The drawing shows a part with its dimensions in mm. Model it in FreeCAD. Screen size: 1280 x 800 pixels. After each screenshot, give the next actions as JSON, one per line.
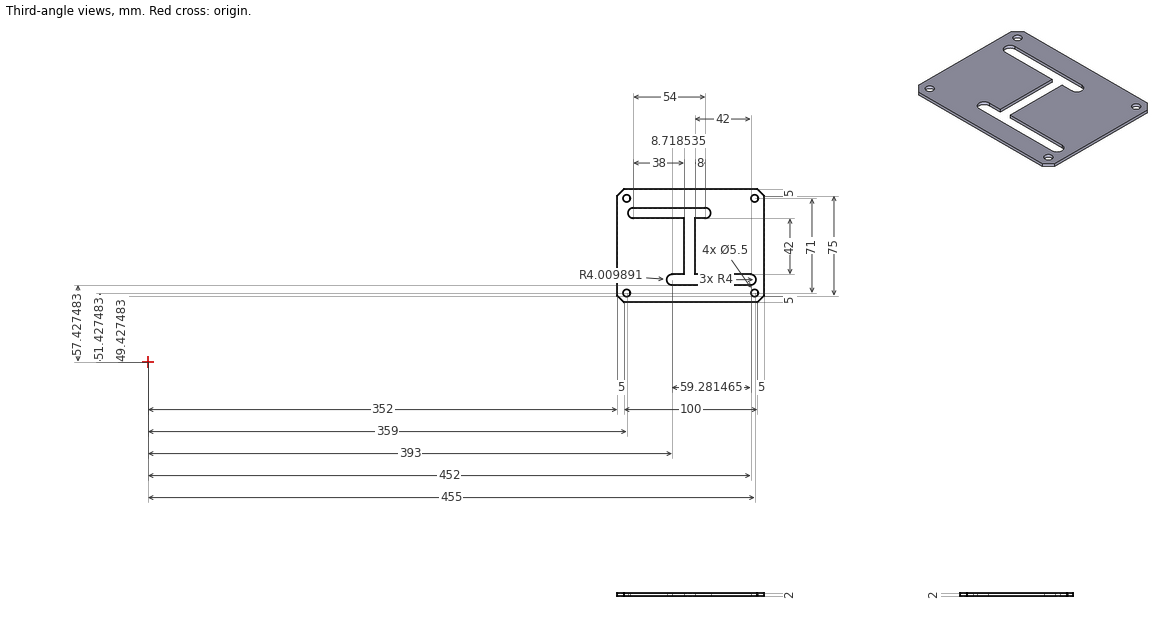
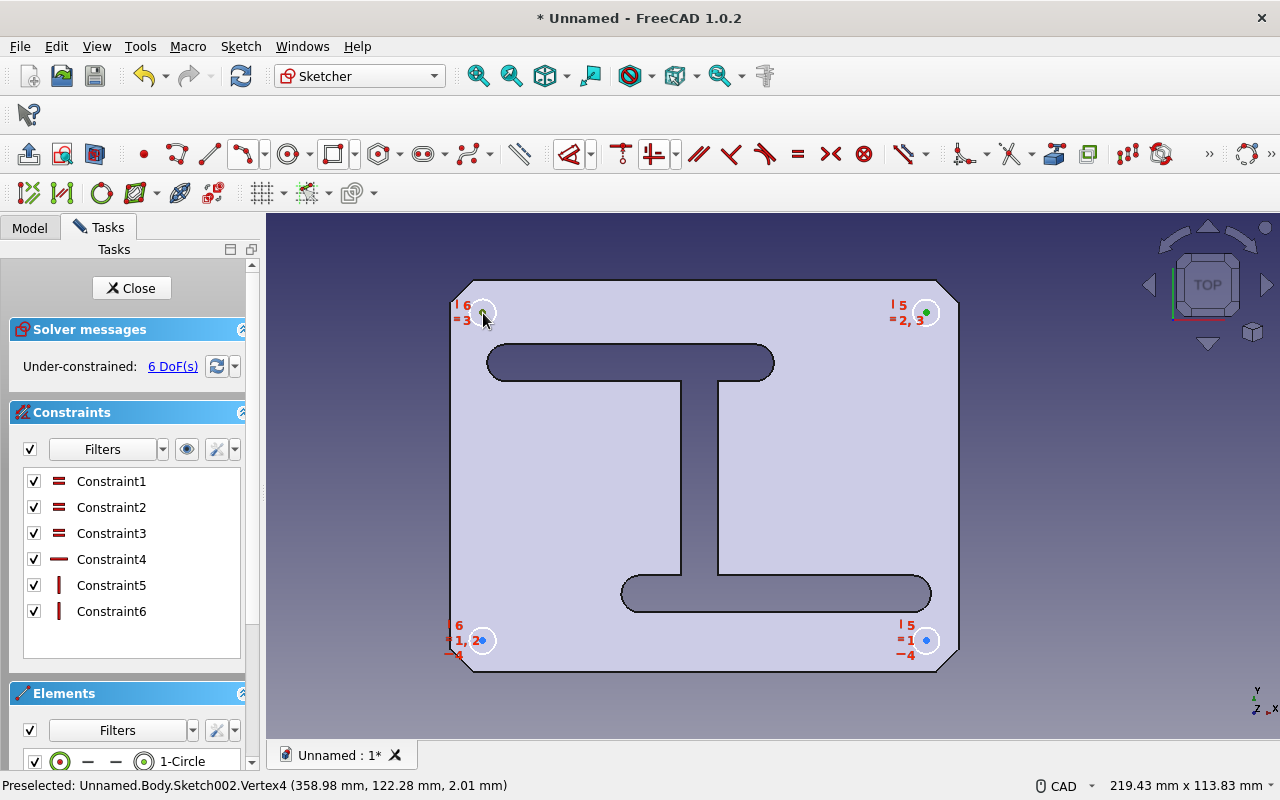
{"action": "left_click", "coordinate": [676, 154]}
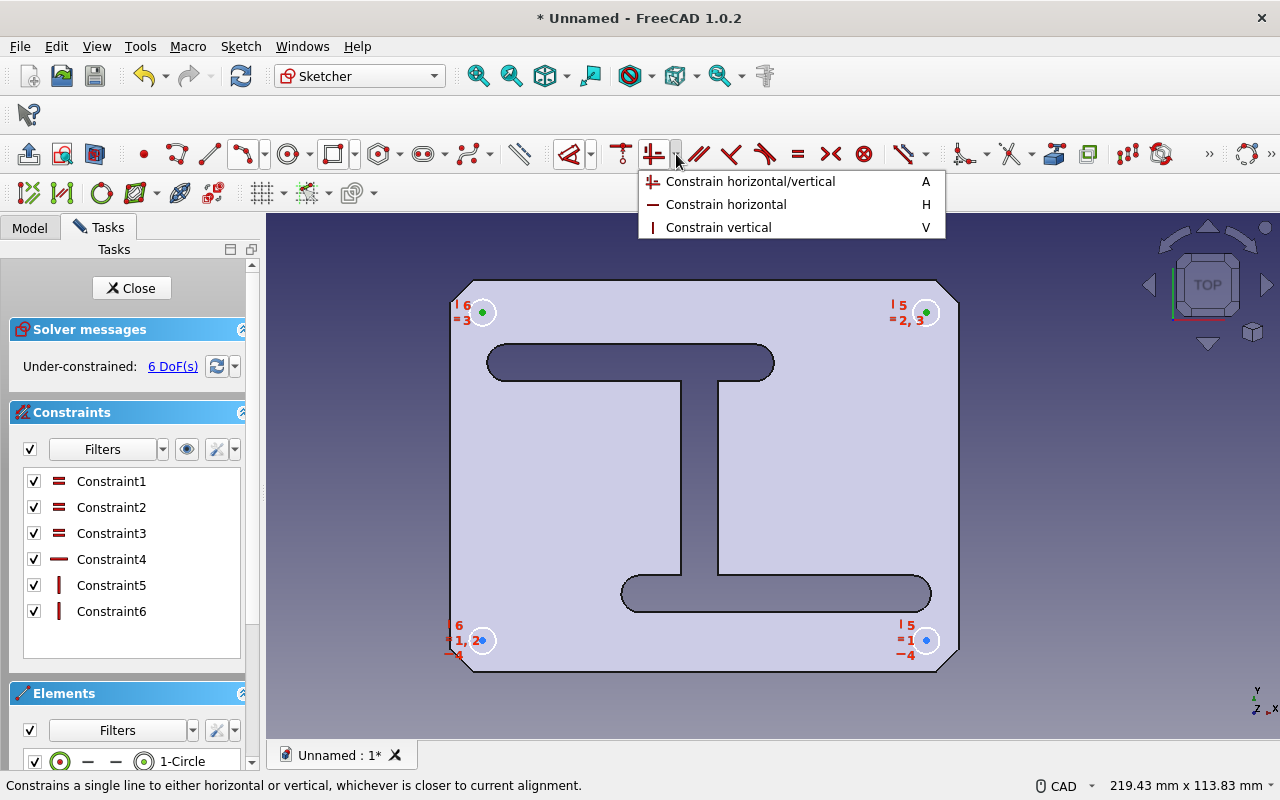
{"action": "left_click", "coordinate": [792, 204]}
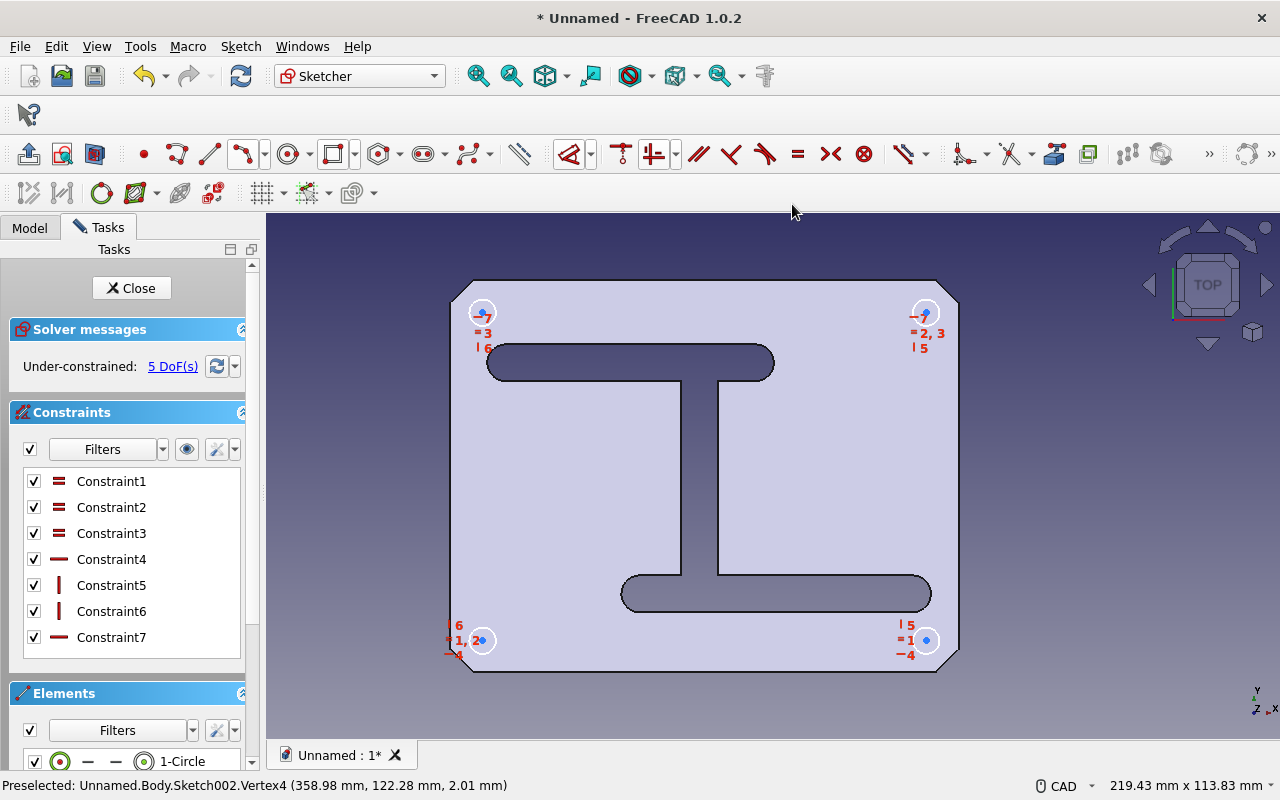
{"action": "scroll", "coordinate": [936, 631], "scroll_direction": "up", "scroll_amount": 3}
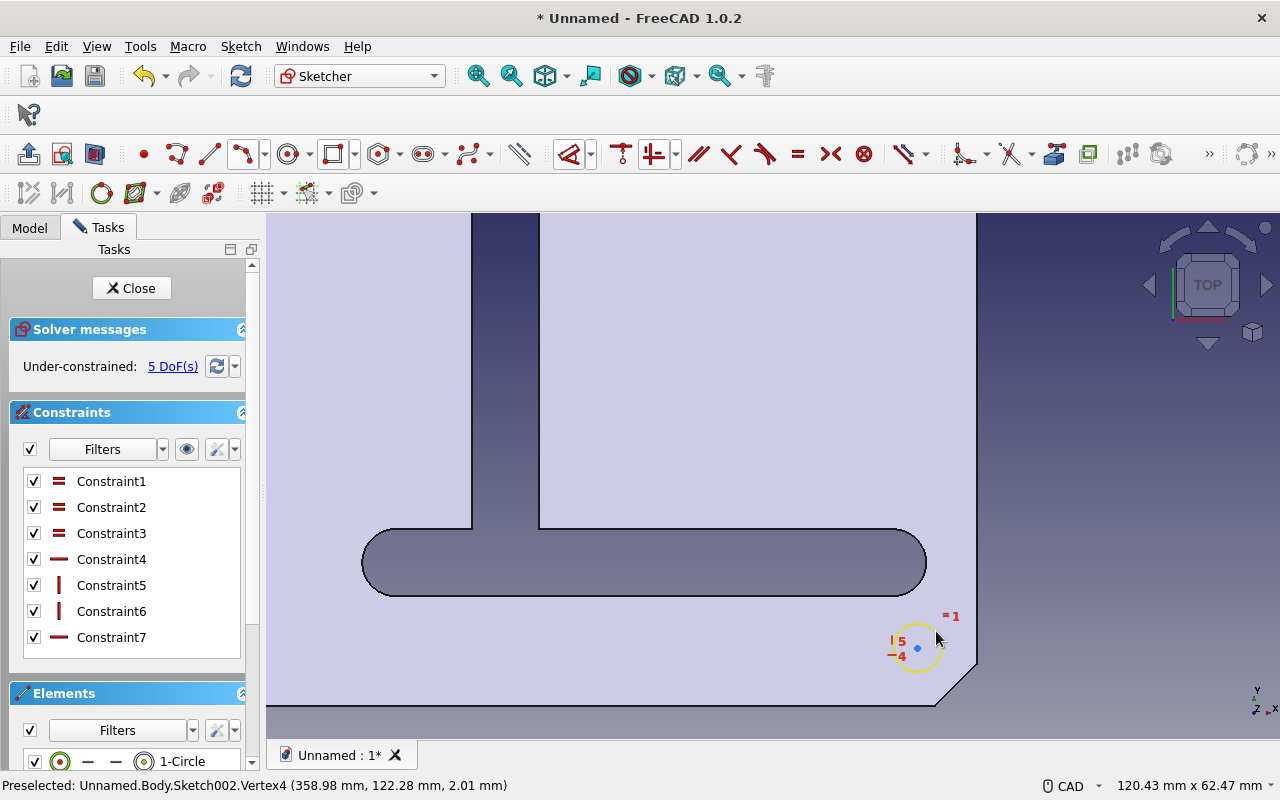
{"action": "left_click", "coordinate": [935, 631]}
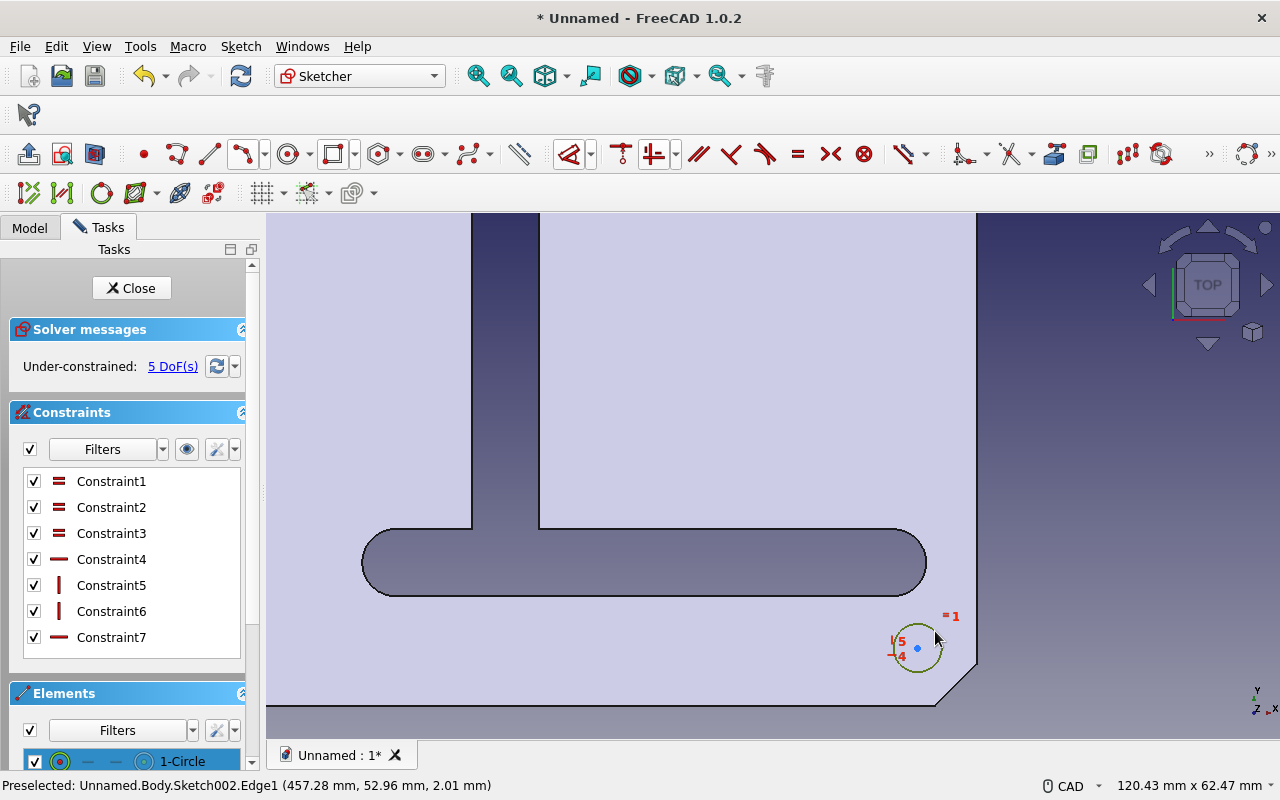
{"action": "left_click", "coordinate": [590, 154]}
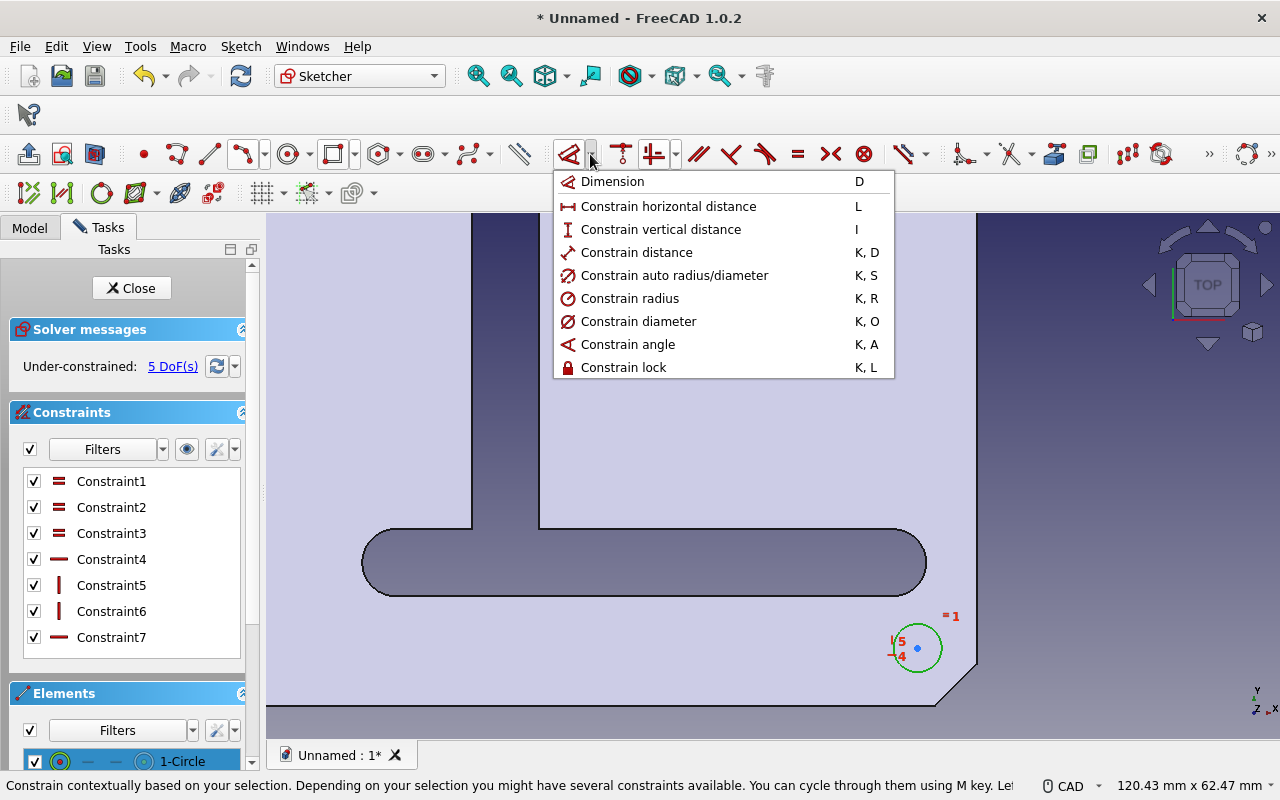
{"action": "left_click", "coordinate": [724, 322]}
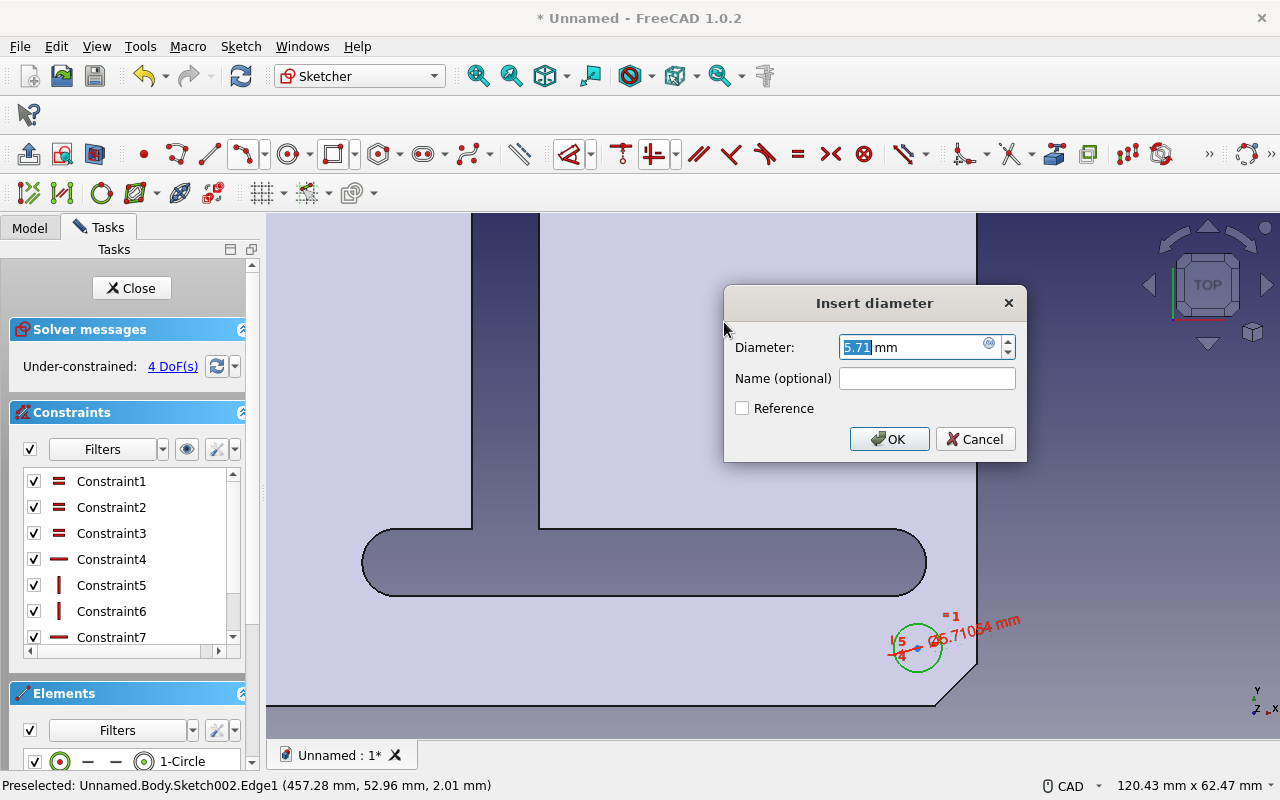
{"action": "type", "text": "5.5"}
{"action": "key", "text": "Return"}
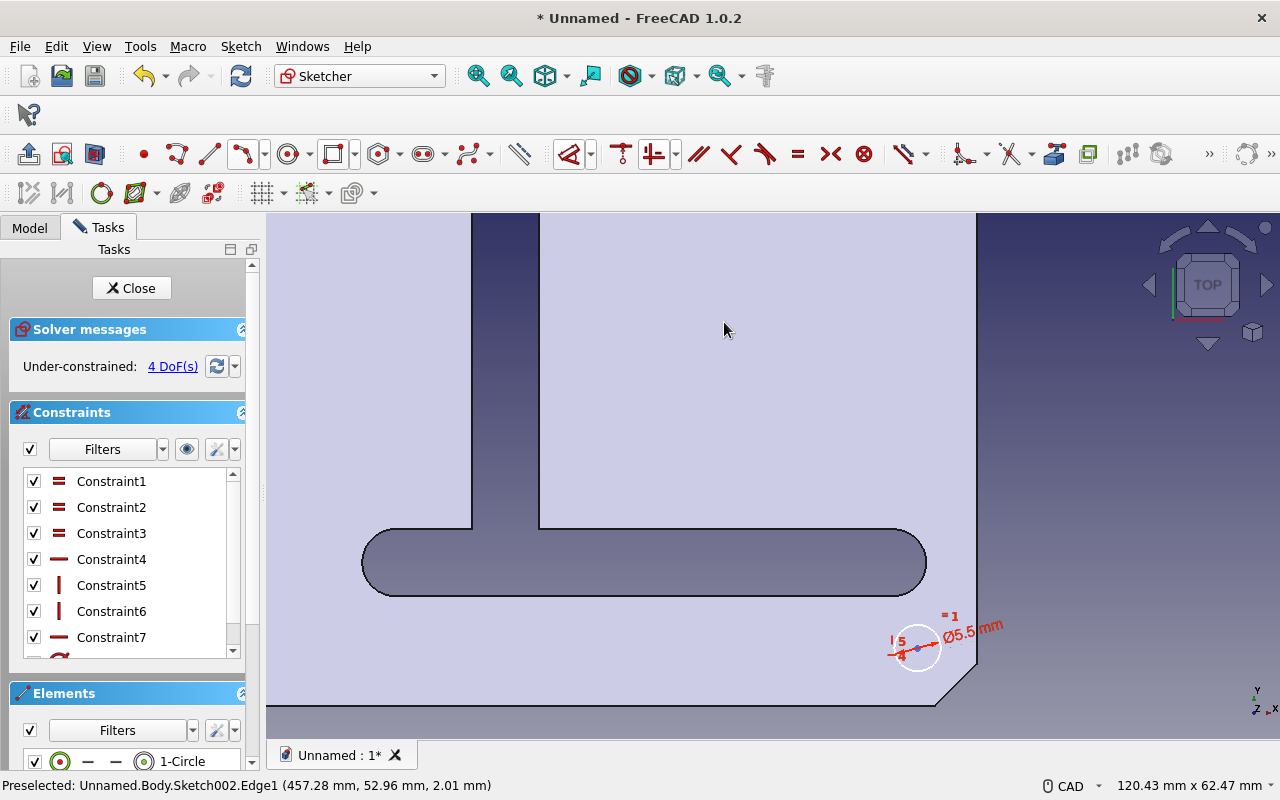
{"action": "left_click", "coordinate": [918, 648]}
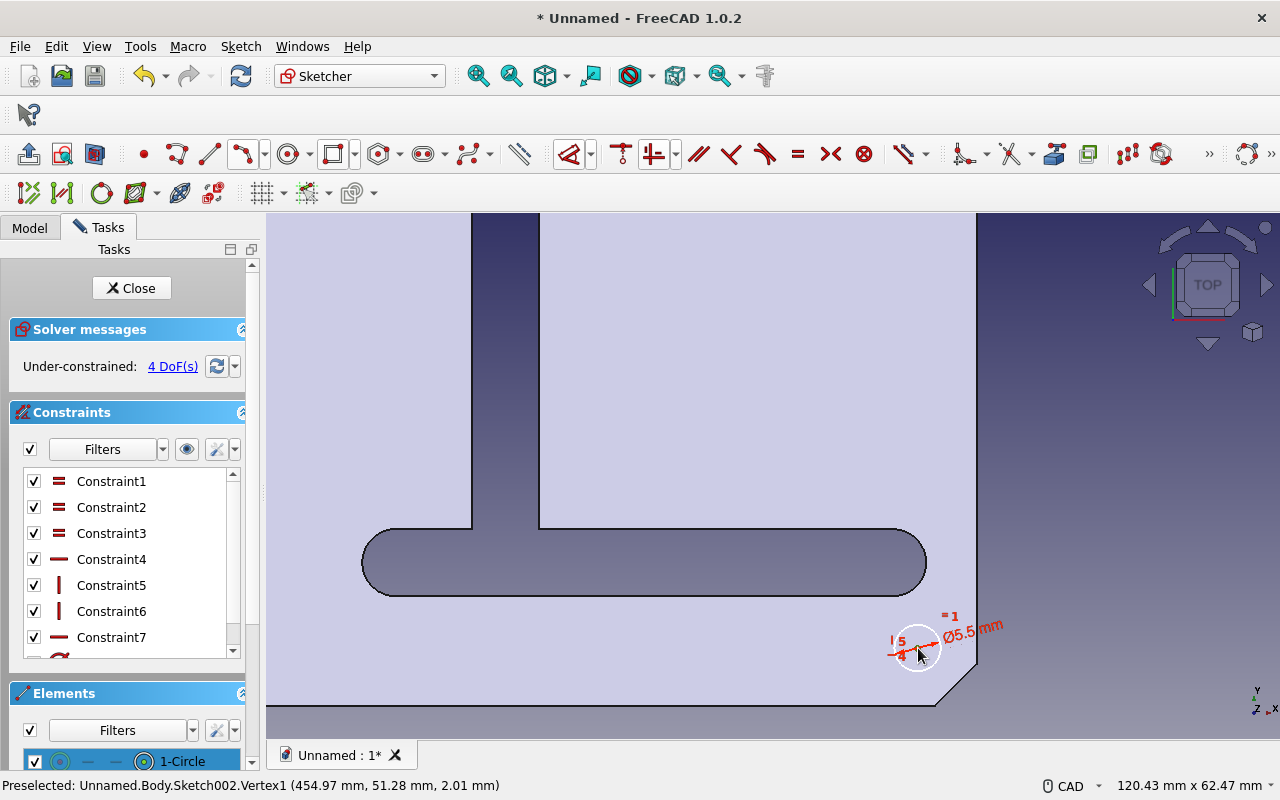
{"action": "left_click", "coordinate": [590, 154]}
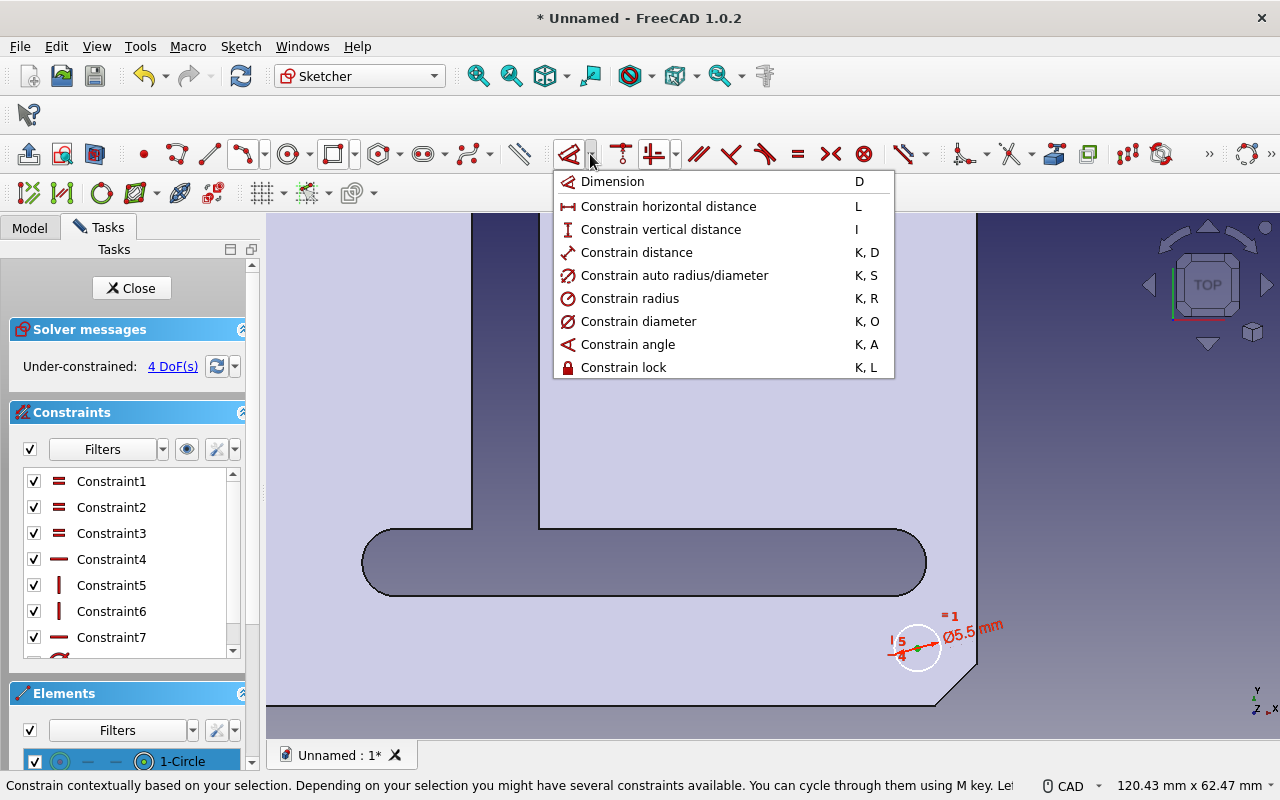
{"action": "left_click", "coordinate": [724, 206]}